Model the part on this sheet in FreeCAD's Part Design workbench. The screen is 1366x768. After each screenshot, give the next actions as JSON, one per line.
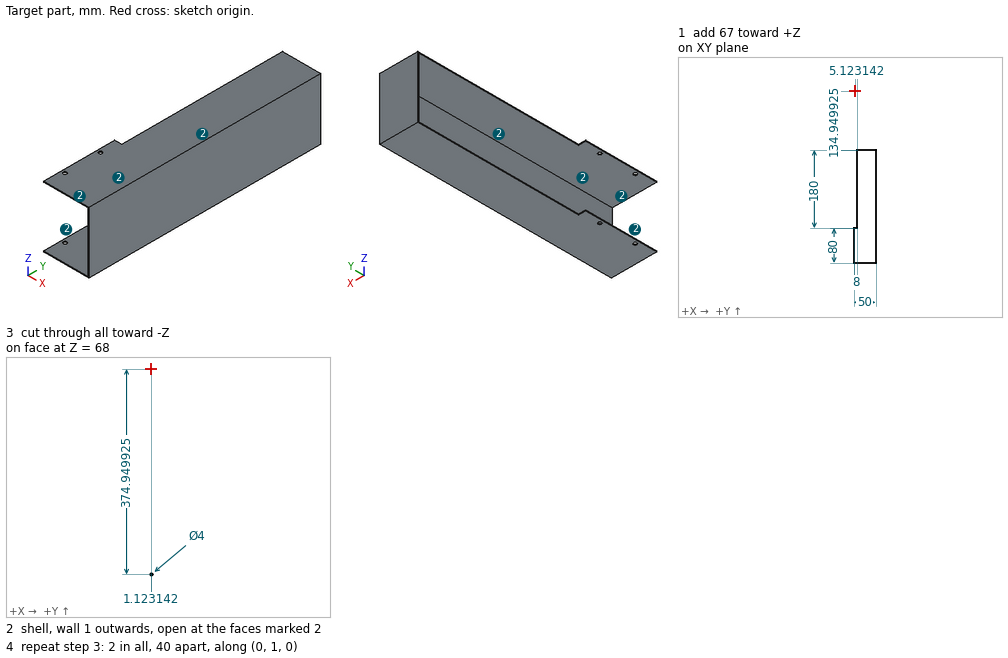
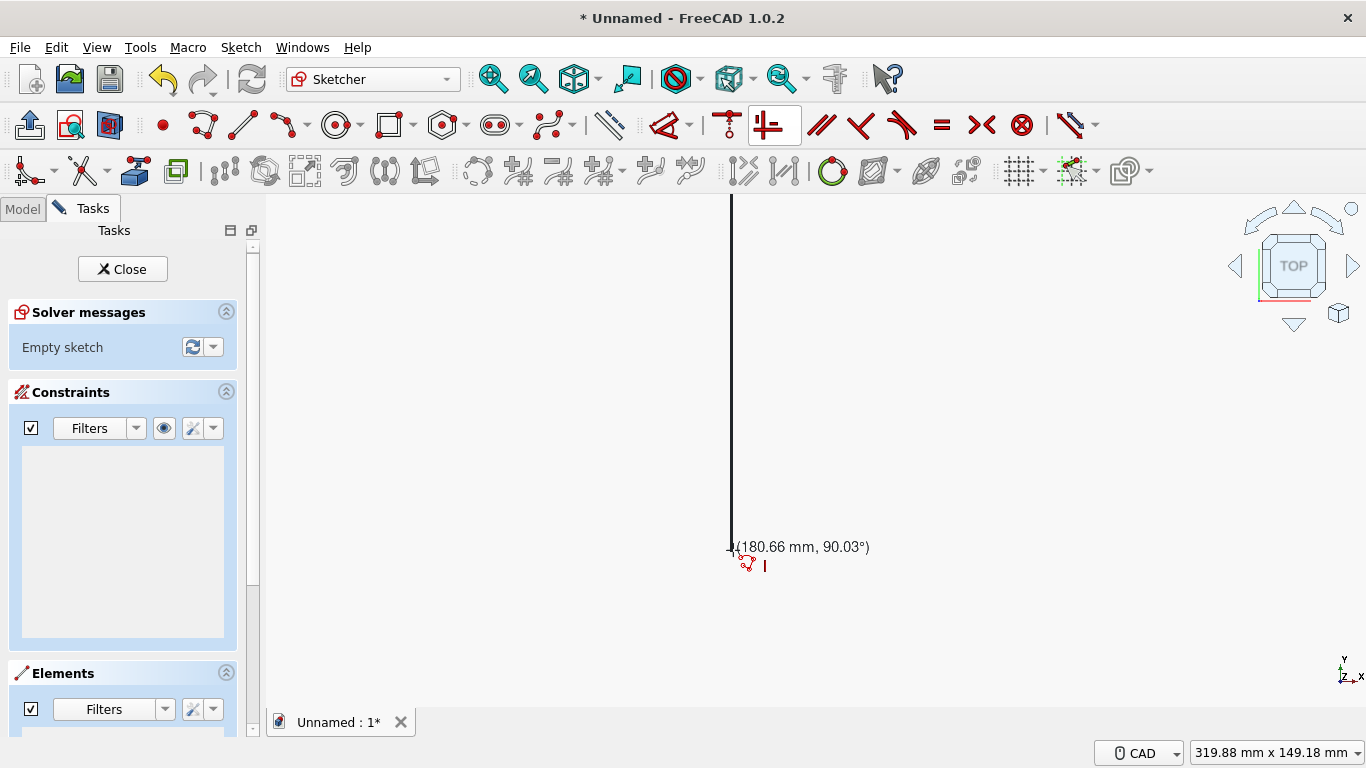
{"action": "left_click", "coordinate": [732, 549]}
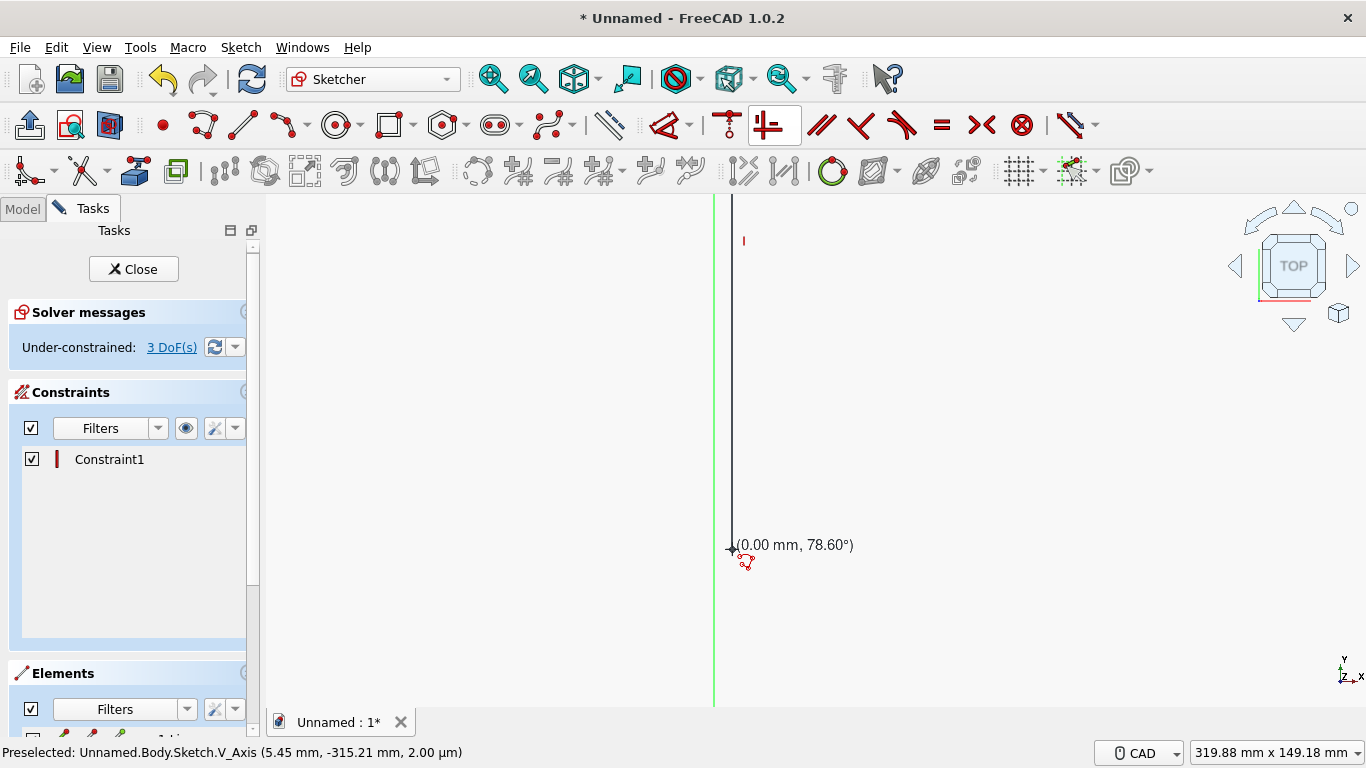
{"action": "scroll", "coordinate": [704, 549], "scroll_direction": "up", "scroll_amount": 3}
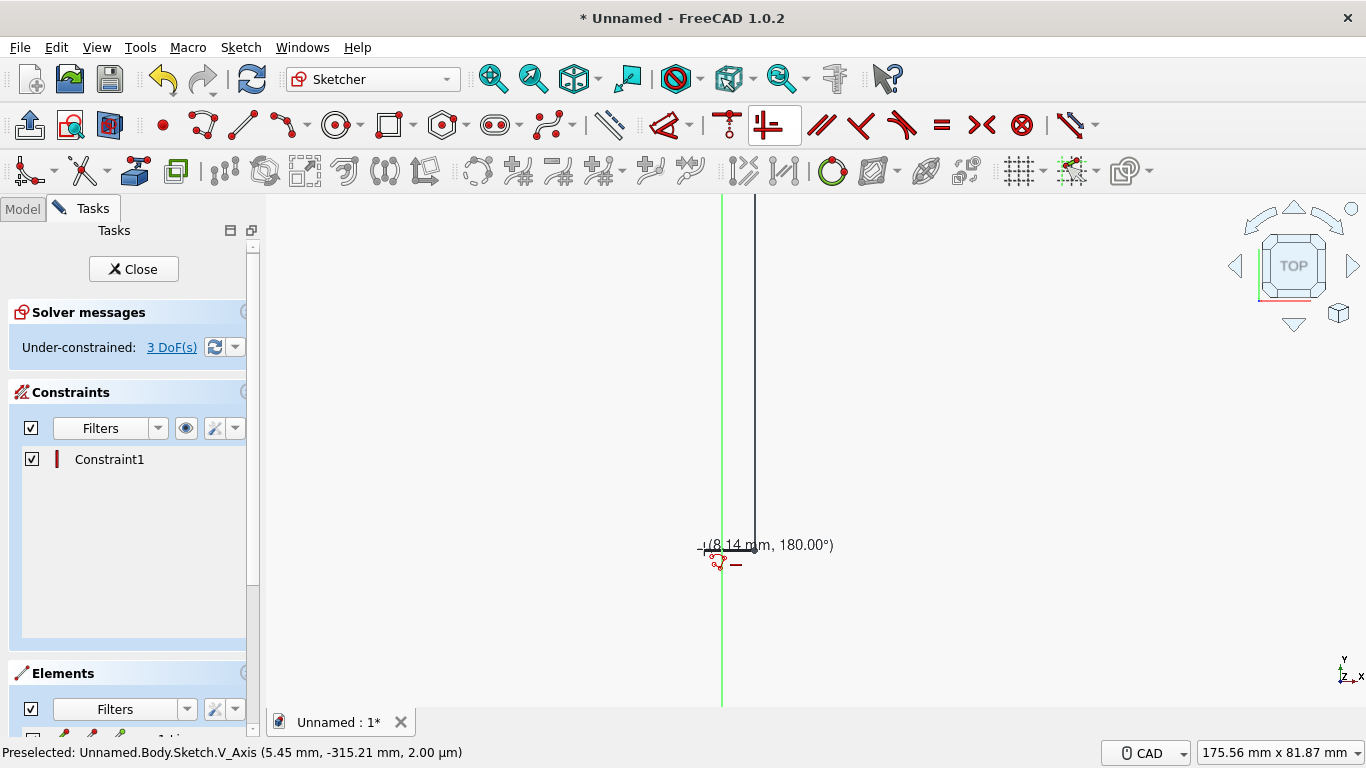
{"action": "left_click", "coordinate": [704, 548]}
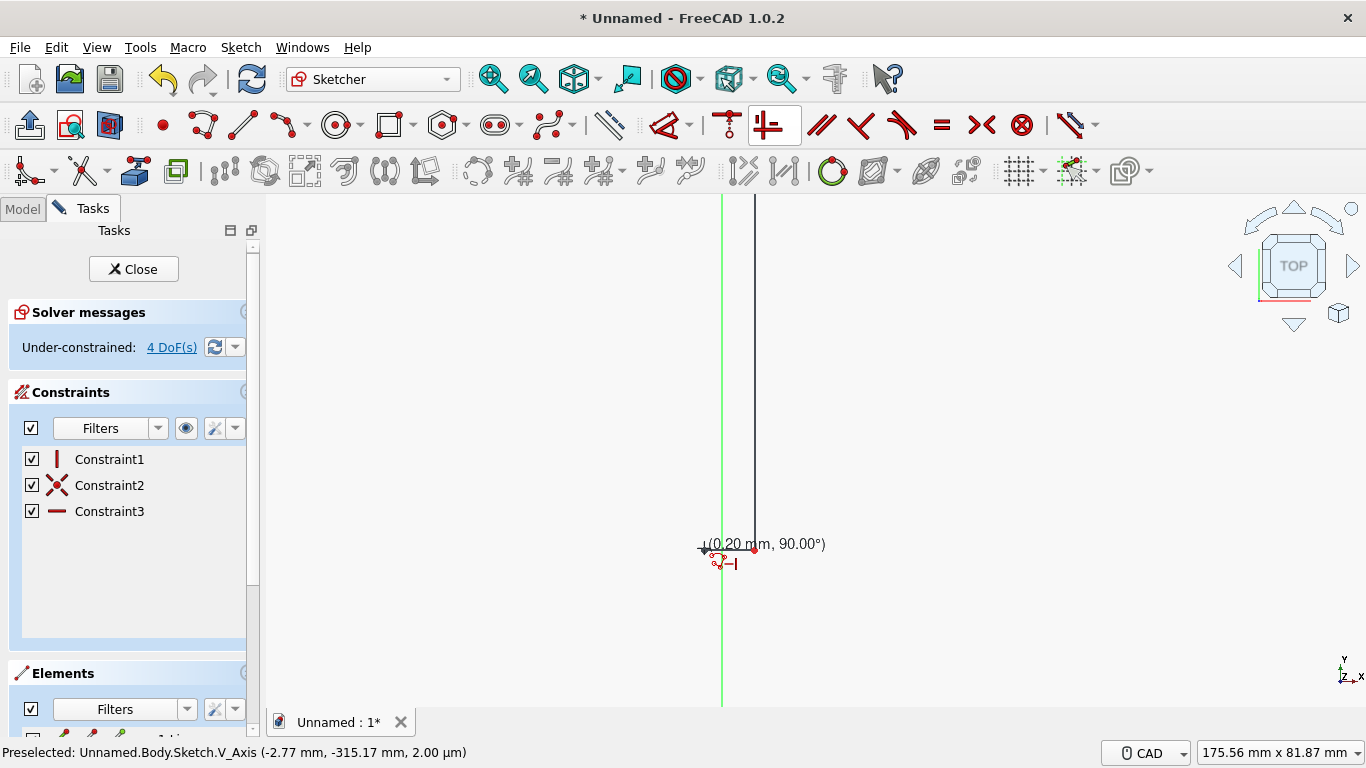
{"action": "scroll", "coordinate": [730, 550], "scroll_direction": "down", "scroll_amount": 10}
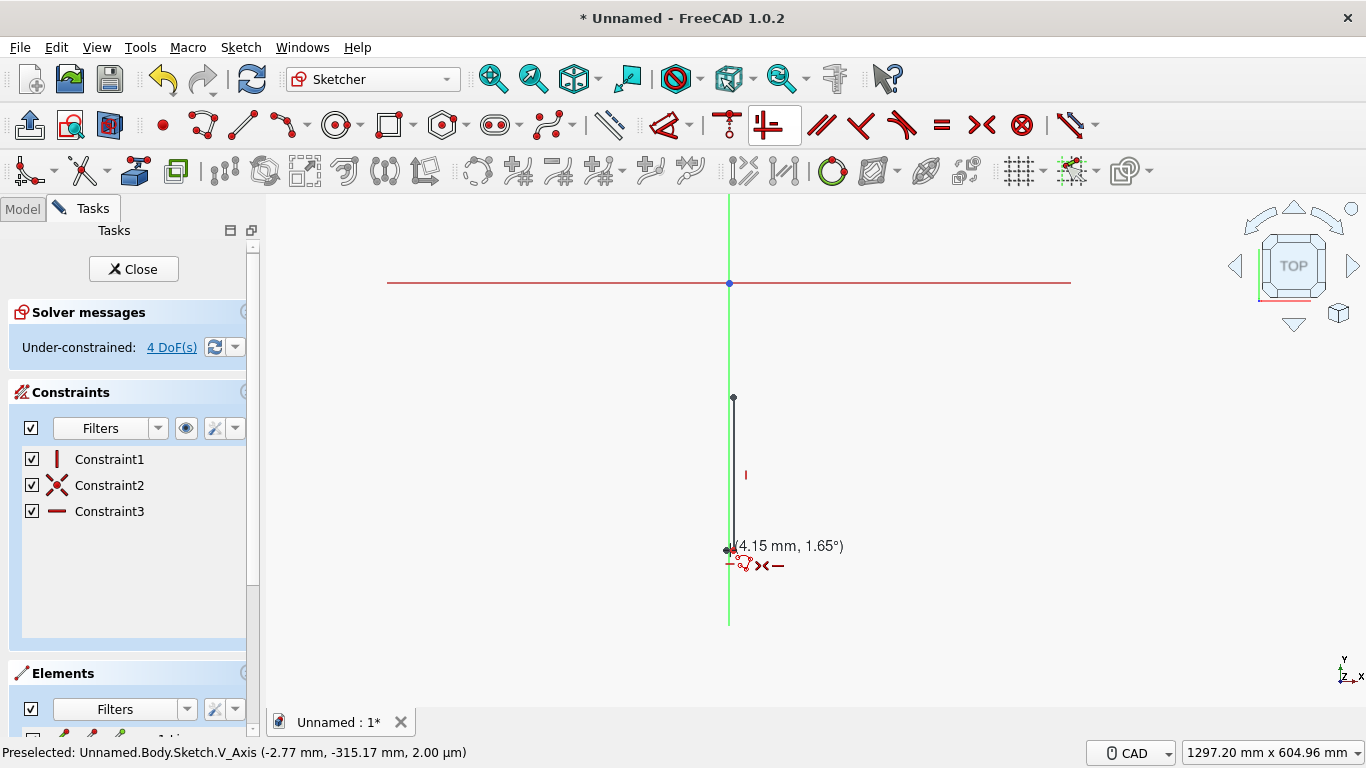
{"action": "scroll", "coordinate": [727, 618], "scroll_direction": "up", "scroll_amount": 10}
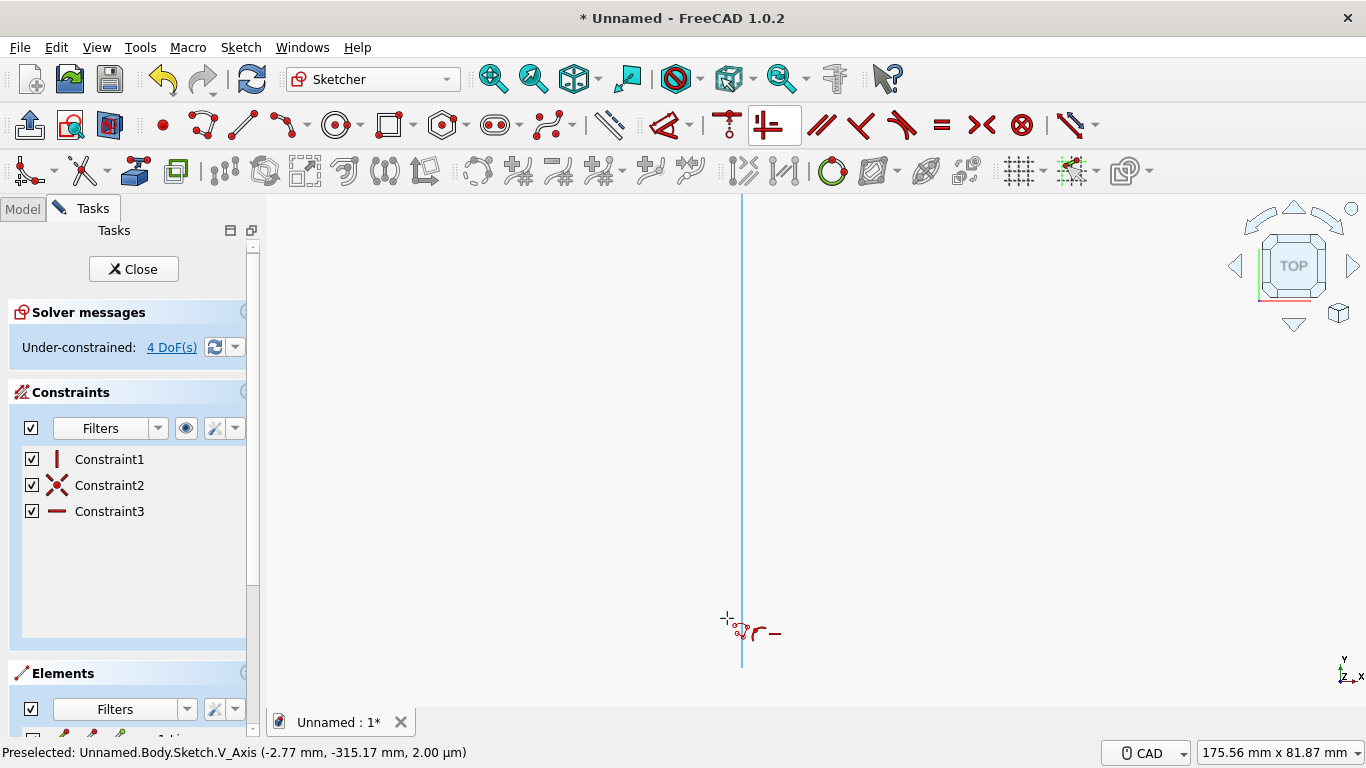
{"action": "left_click", "coordinate": [723, 615]}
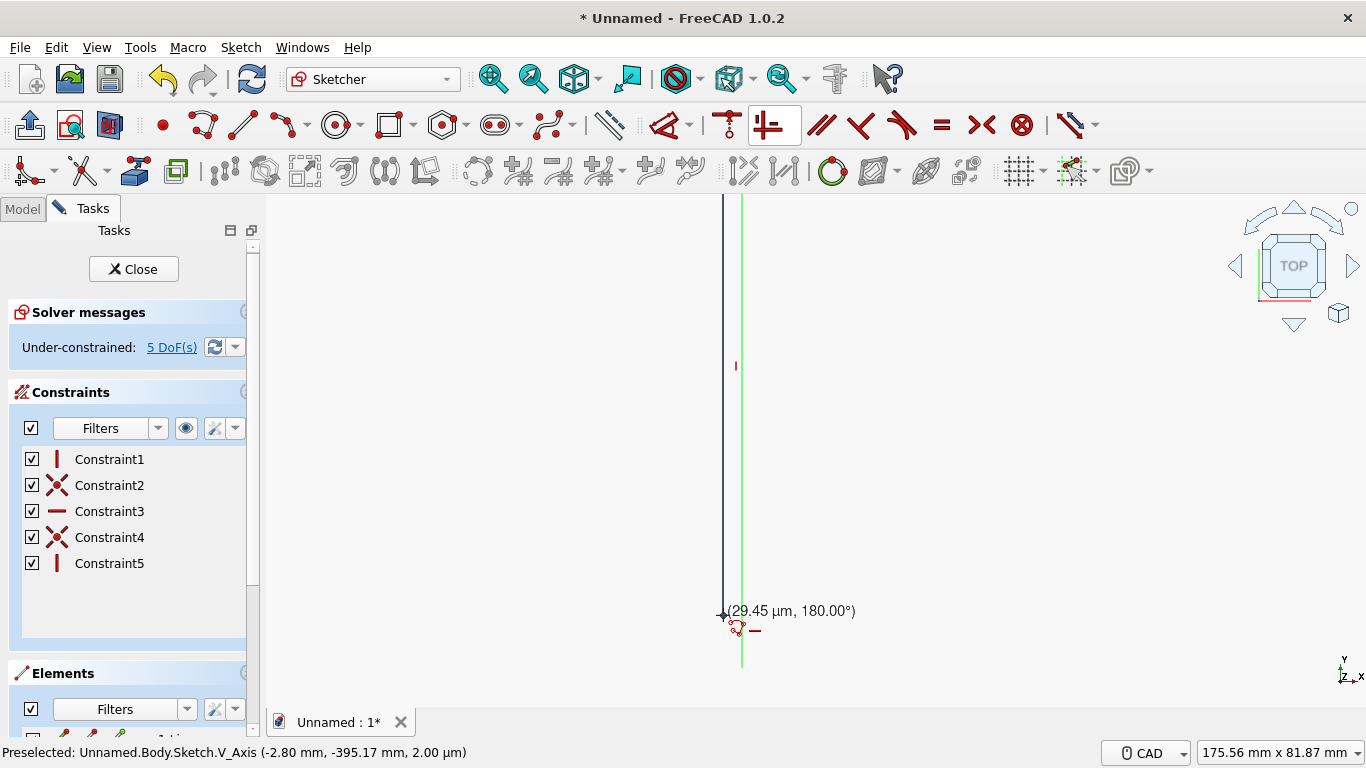
{"action": "scroll", "coordinate": [727, 618], "scroll_direction": "down", "scroll_amount": 10}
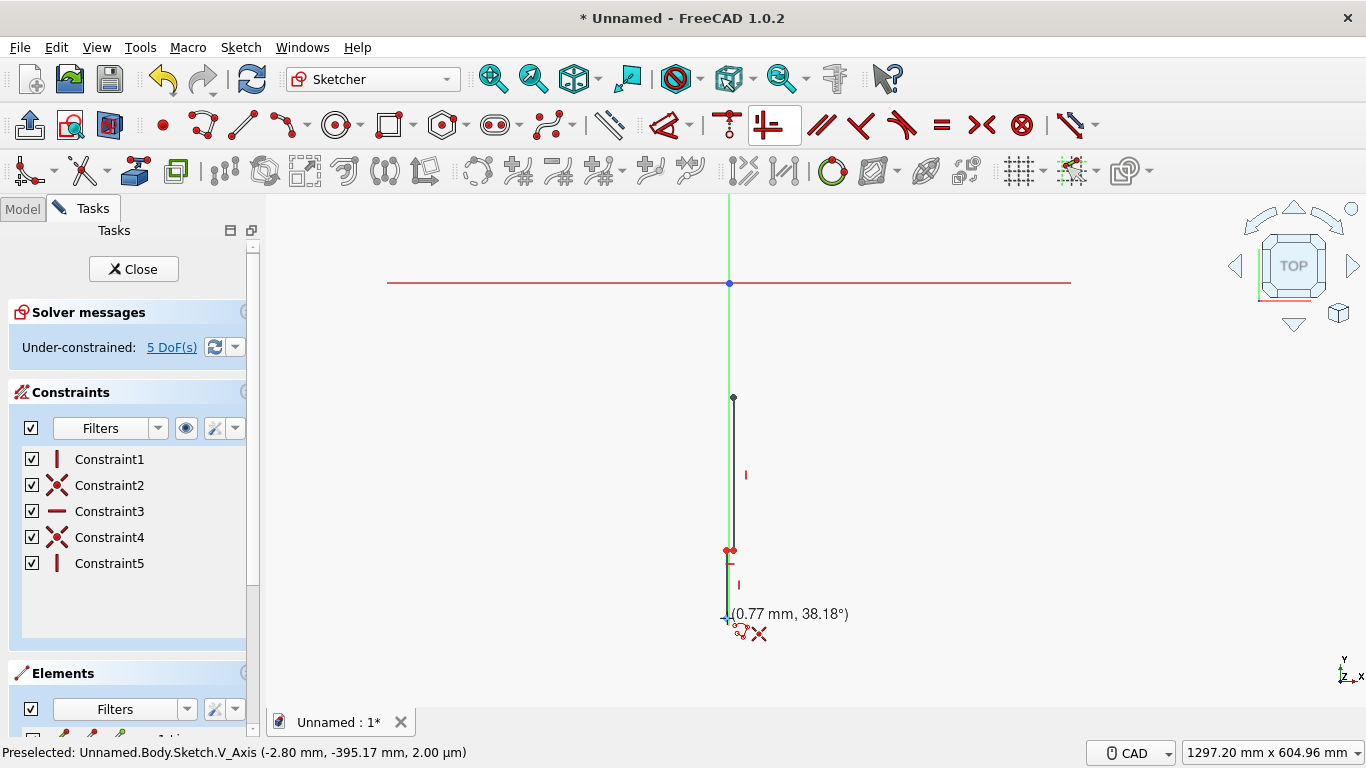
{"action": "left_click", "coordinate": [769, 618]}
{"action": "left_click", "coordinate": [769, 398]}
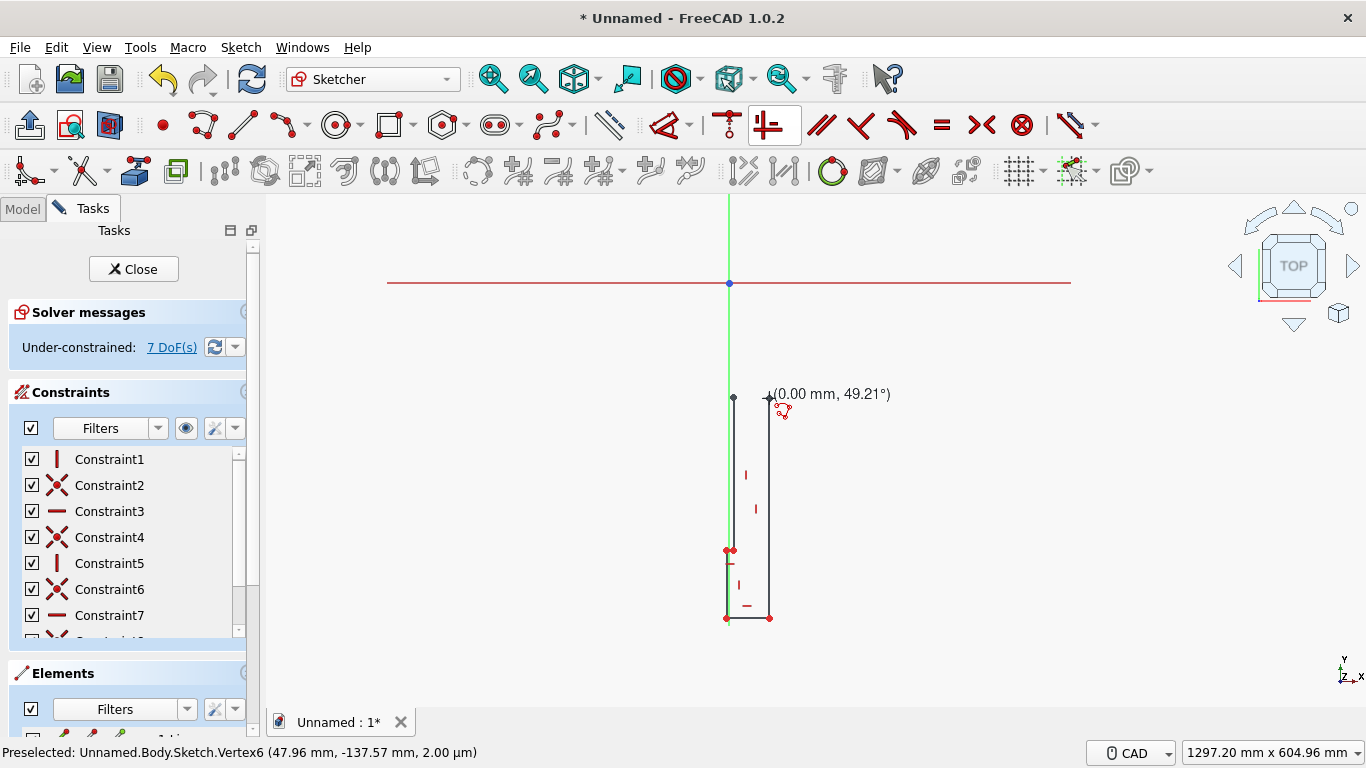
{"action": "scroll", "coordinate": [734, 398], "scroll_direction": "up", "scroll_amount": 7}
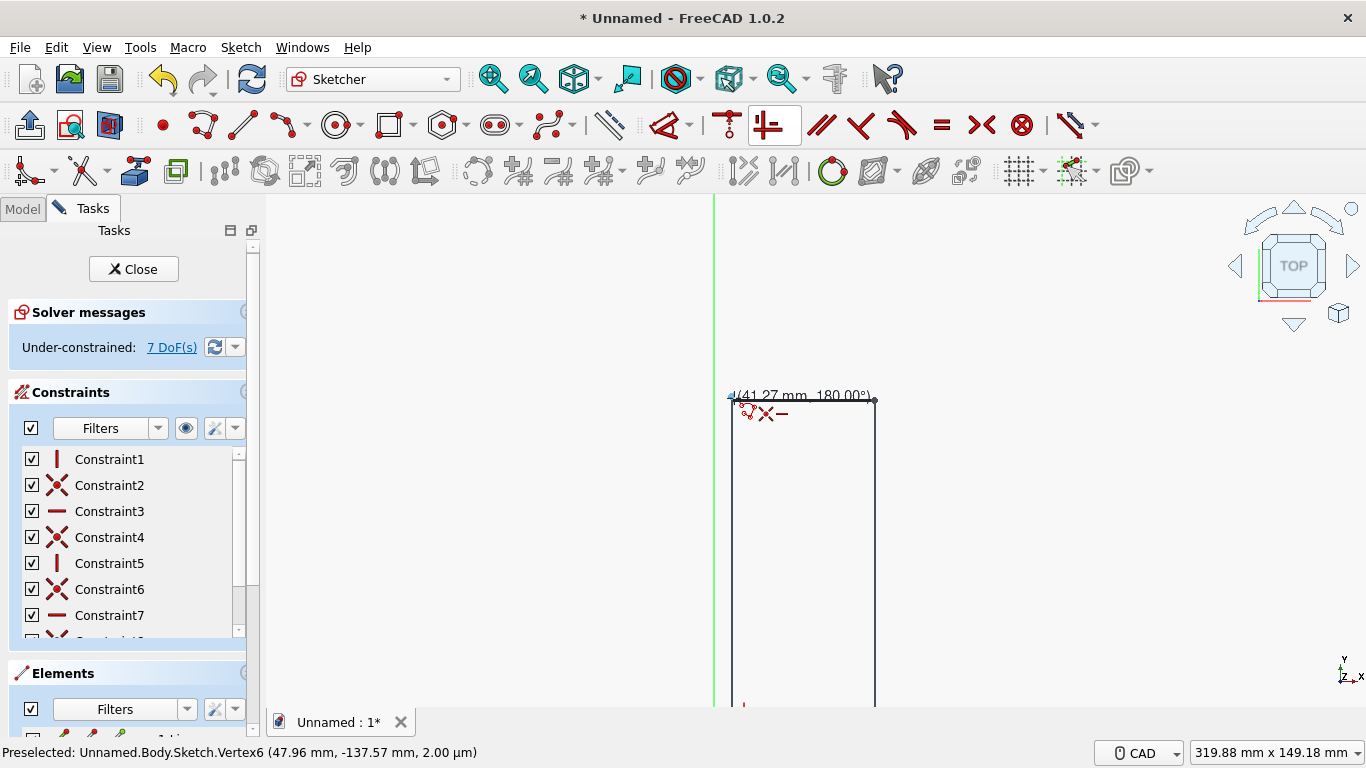
{"action": "left_click", "coordinate": [732, 396]}
{"action": "key", "text": "Escape"}
{"action": "key", "text": "Escape"}